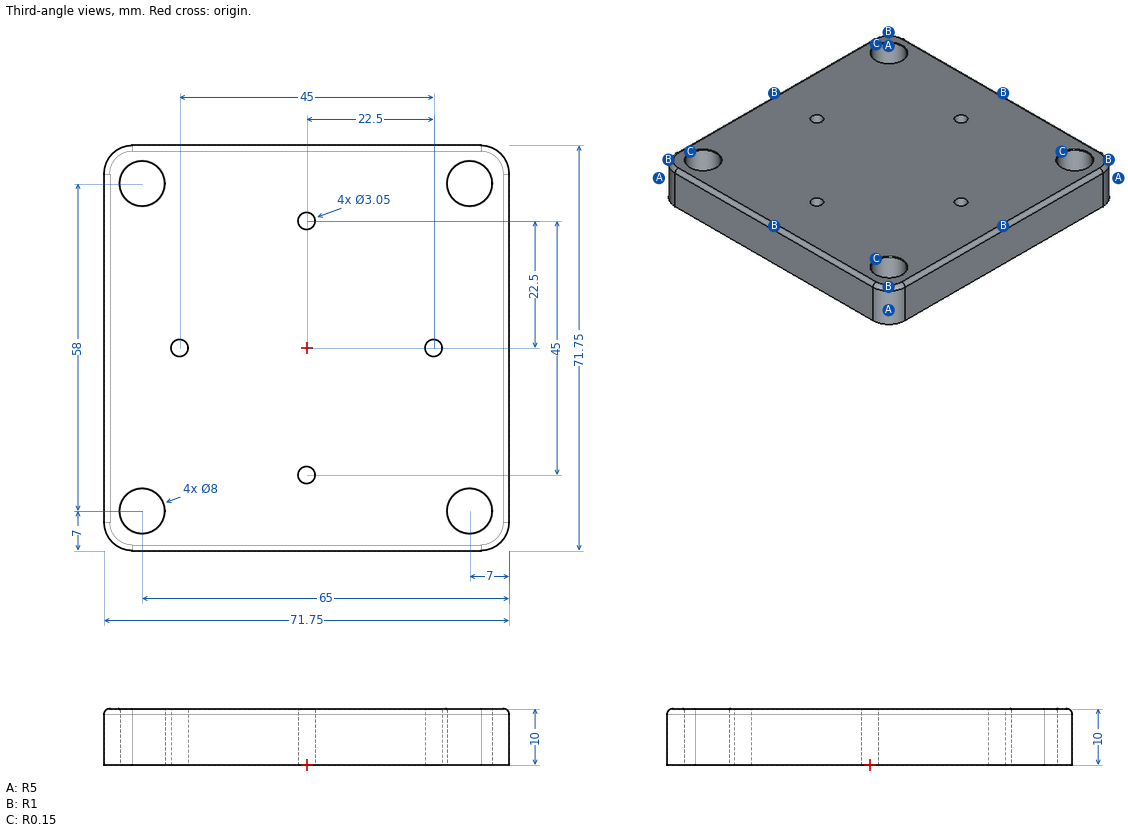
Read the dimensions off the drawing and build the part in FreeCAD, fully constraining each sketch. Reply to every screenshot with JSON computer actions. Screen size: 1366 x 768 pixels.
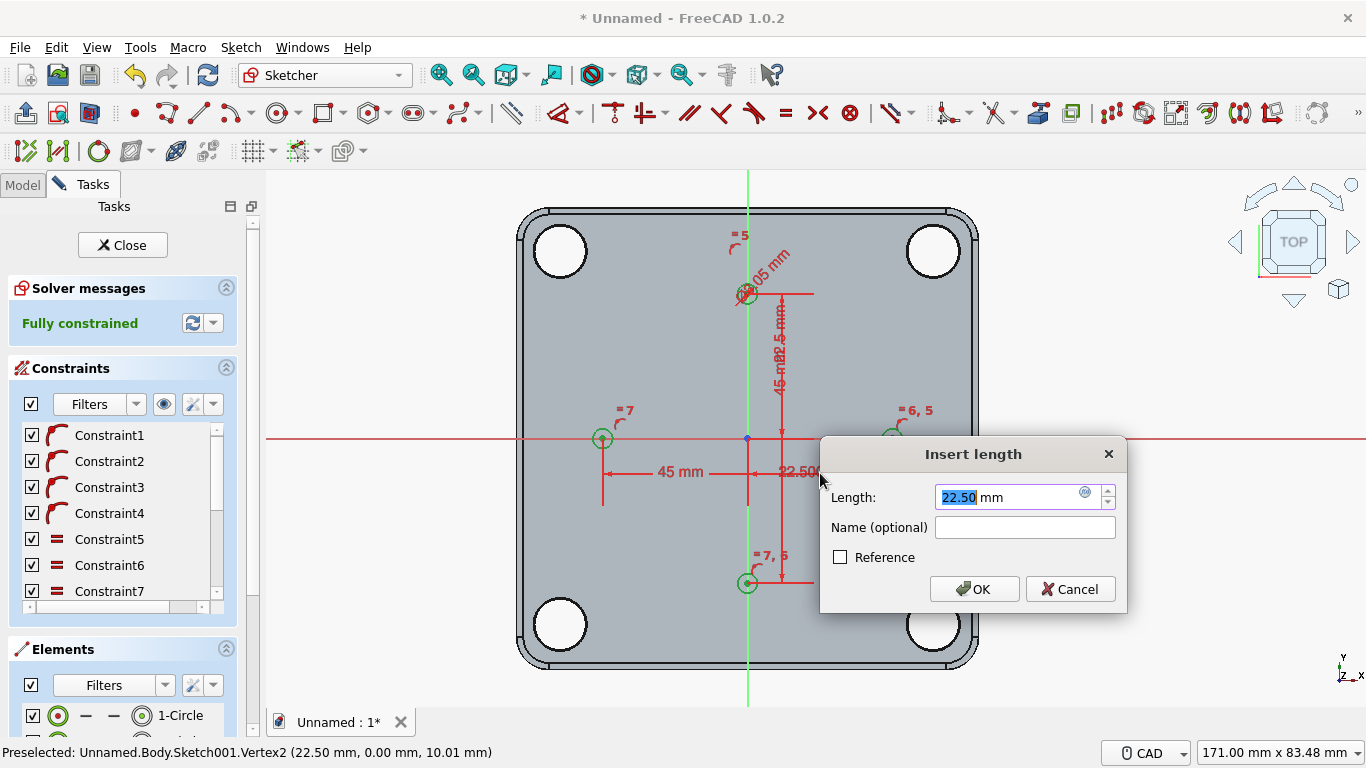
{"action": "type", "text": "22.5"}
{"action": "key", "text": "Return"}
{"action": "key", "text": "Escape"}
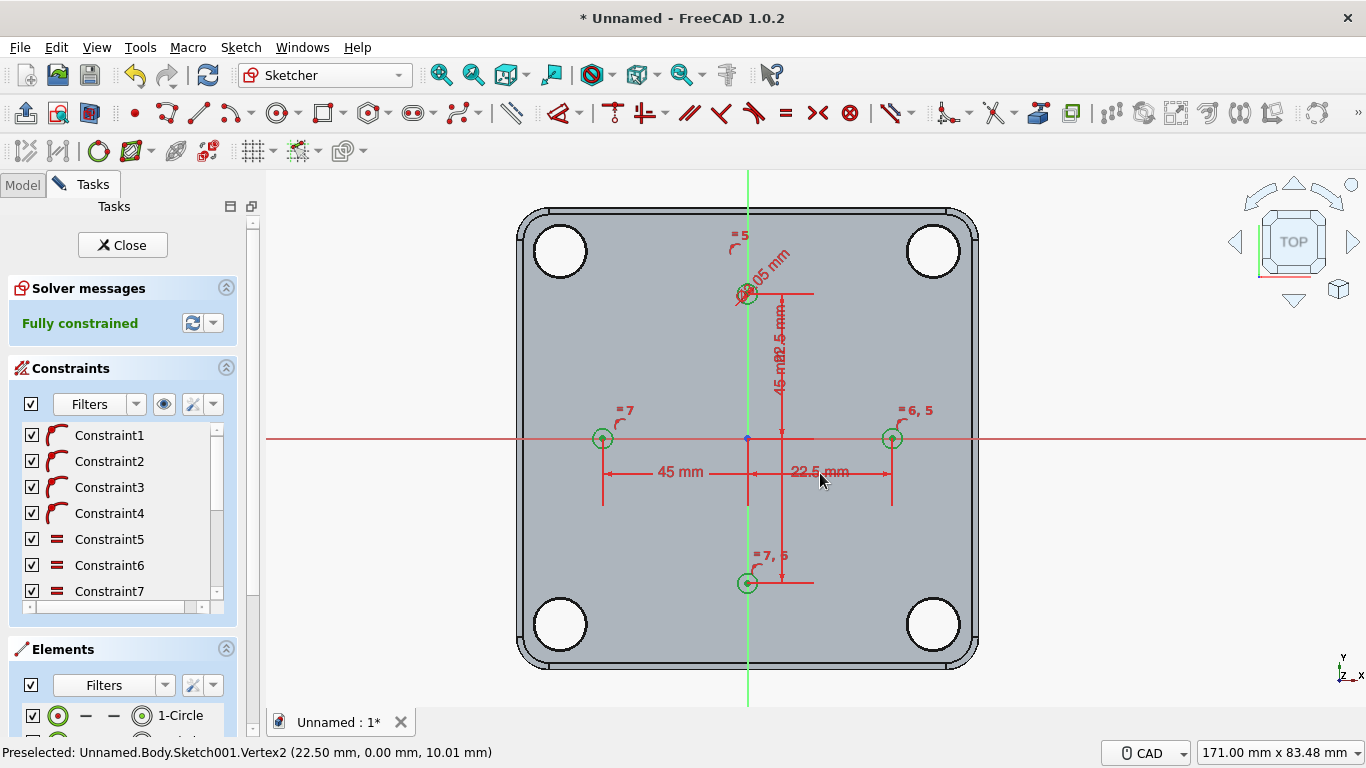
{"action": "left_click", "coordinate": [123, 245]}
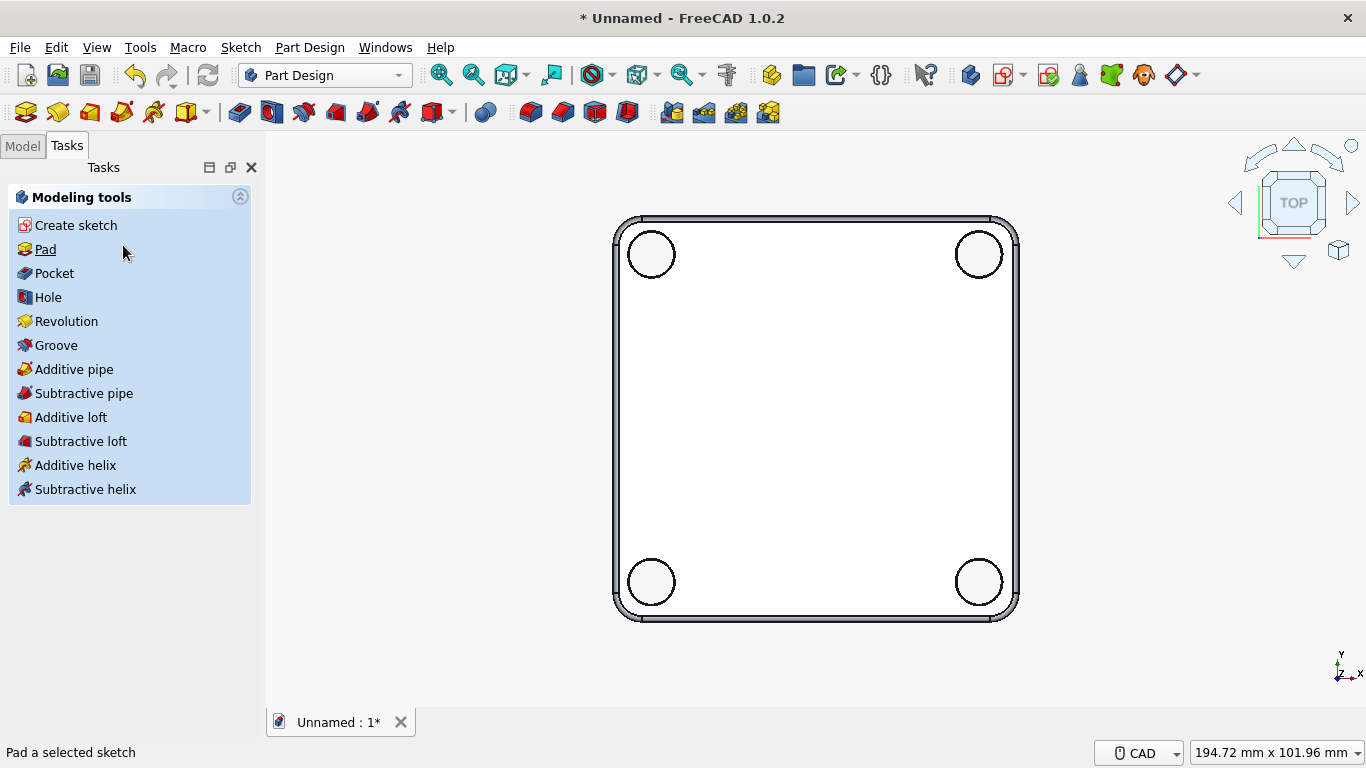
{"action": "left_click", "coordinate": [240, 112]}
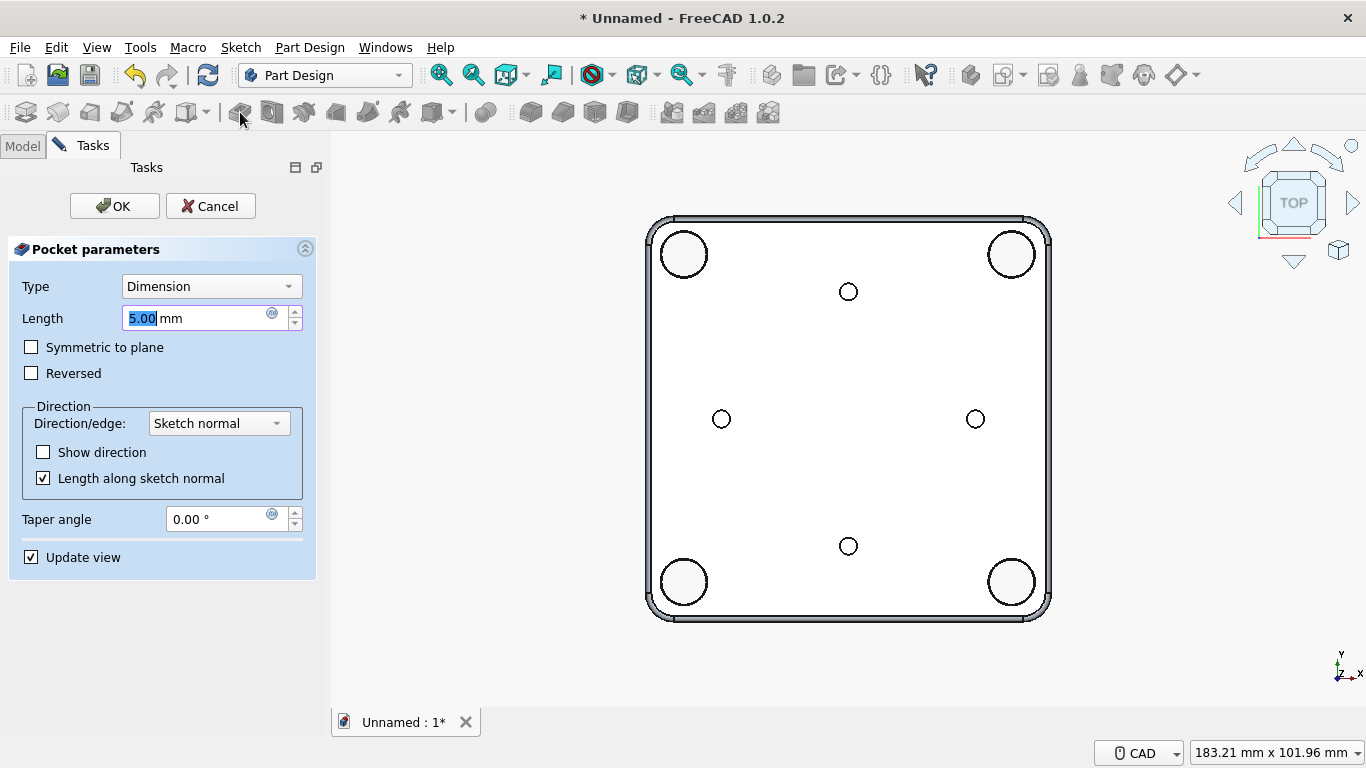
{"action": "type", "text": "10"}
{"action": "key", "text": "Tab"}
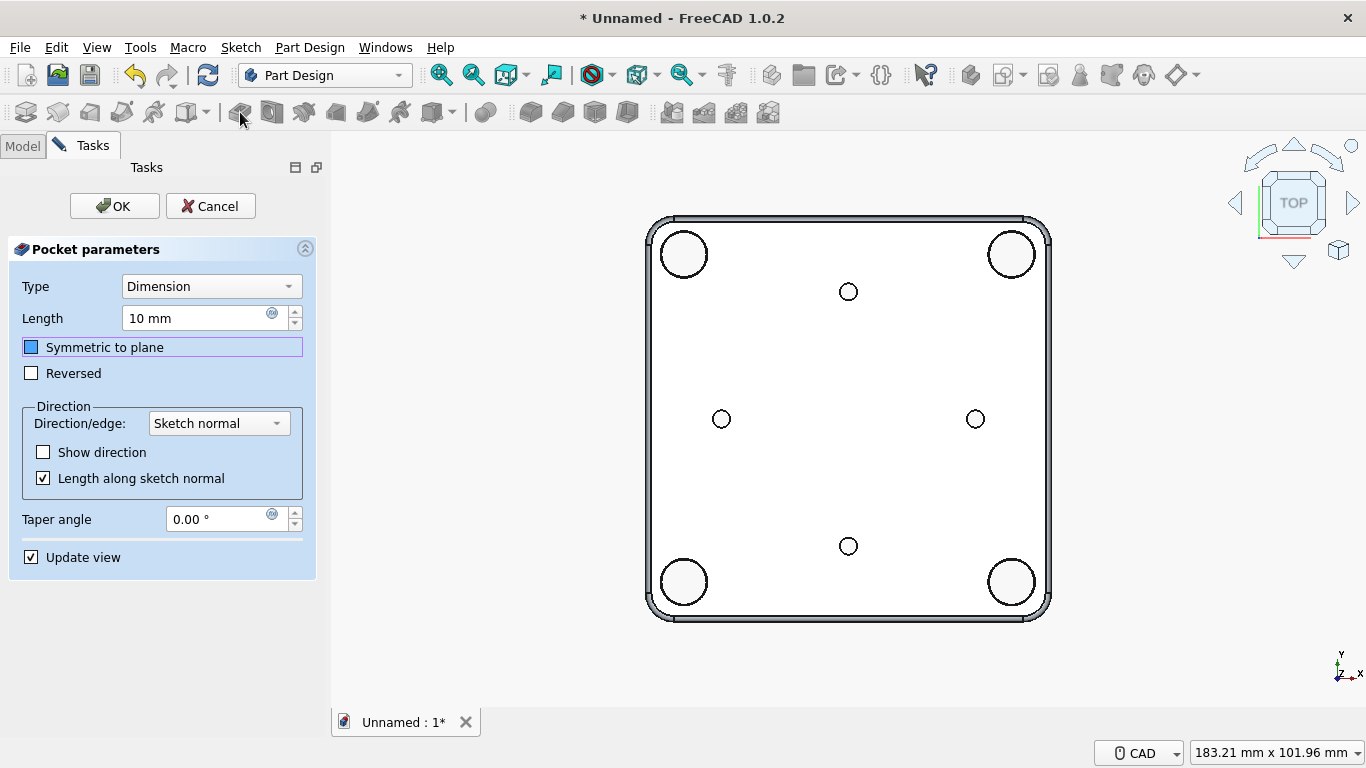
{"action": "left_click", "coordinate": [115, 206]}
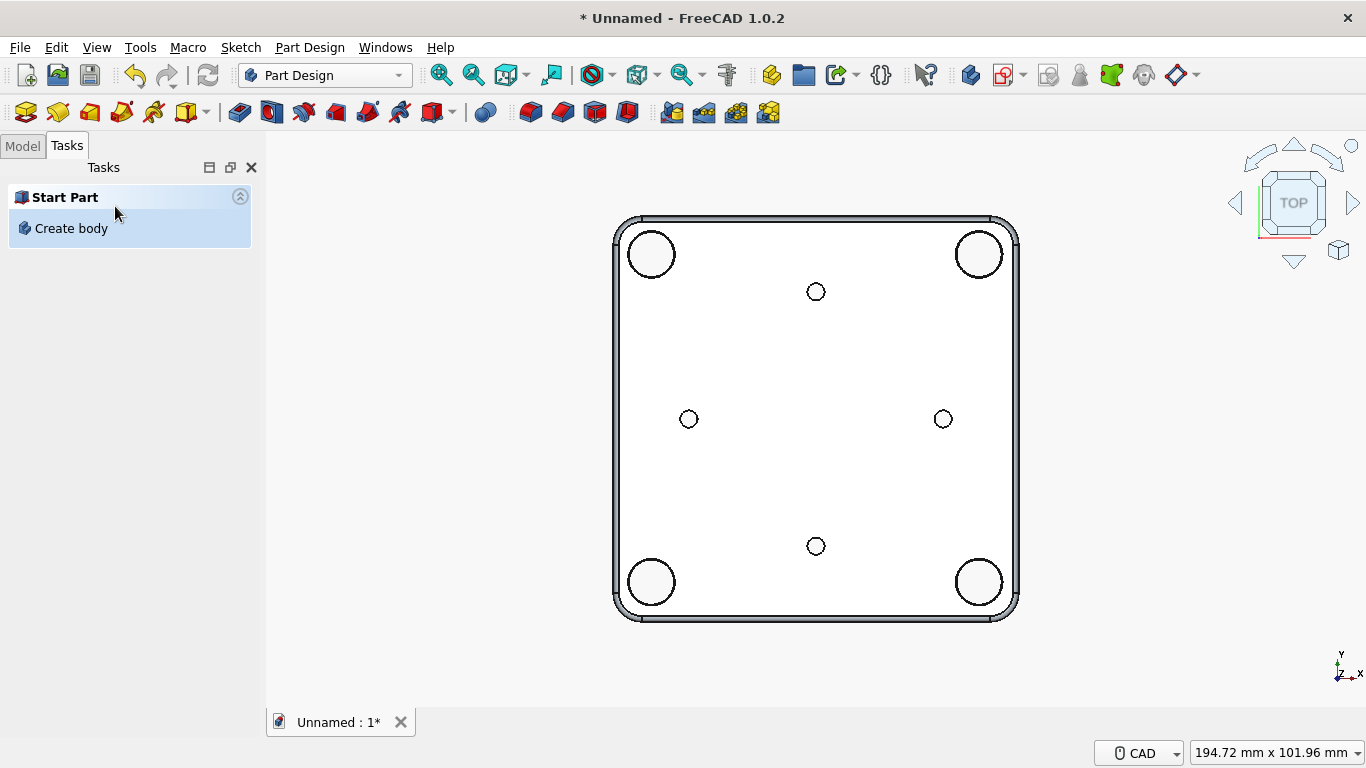
{"action": "key", "text": "0"}